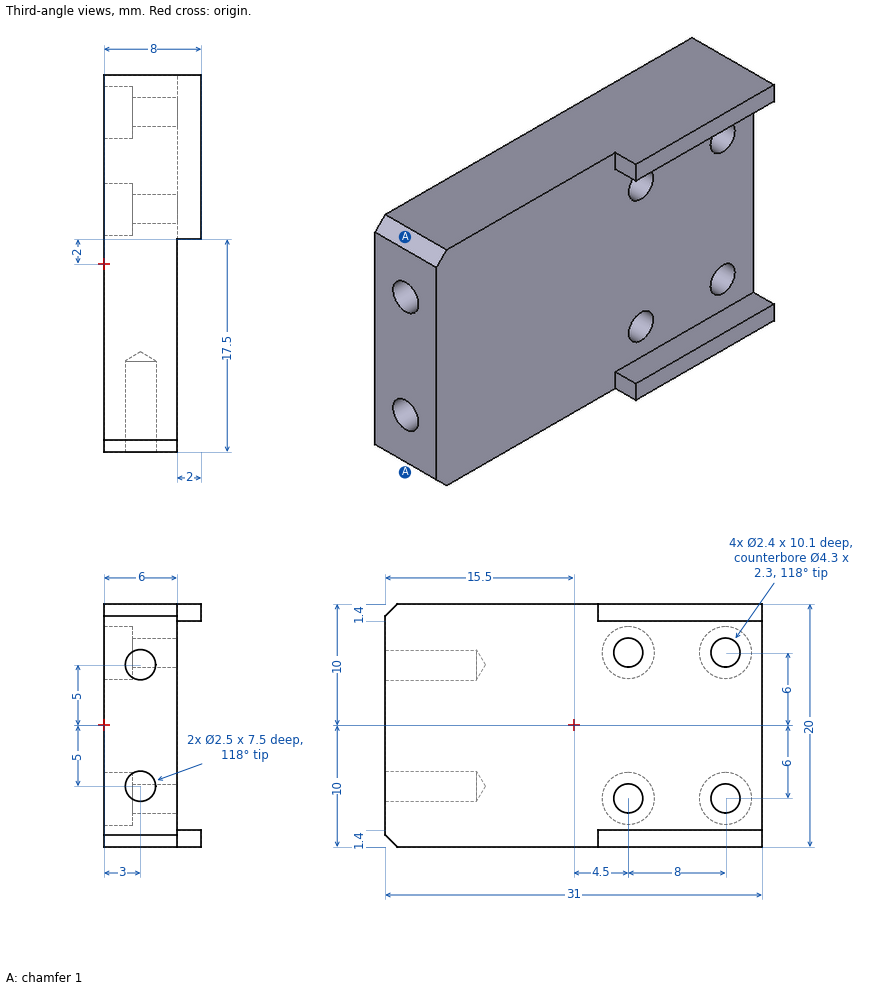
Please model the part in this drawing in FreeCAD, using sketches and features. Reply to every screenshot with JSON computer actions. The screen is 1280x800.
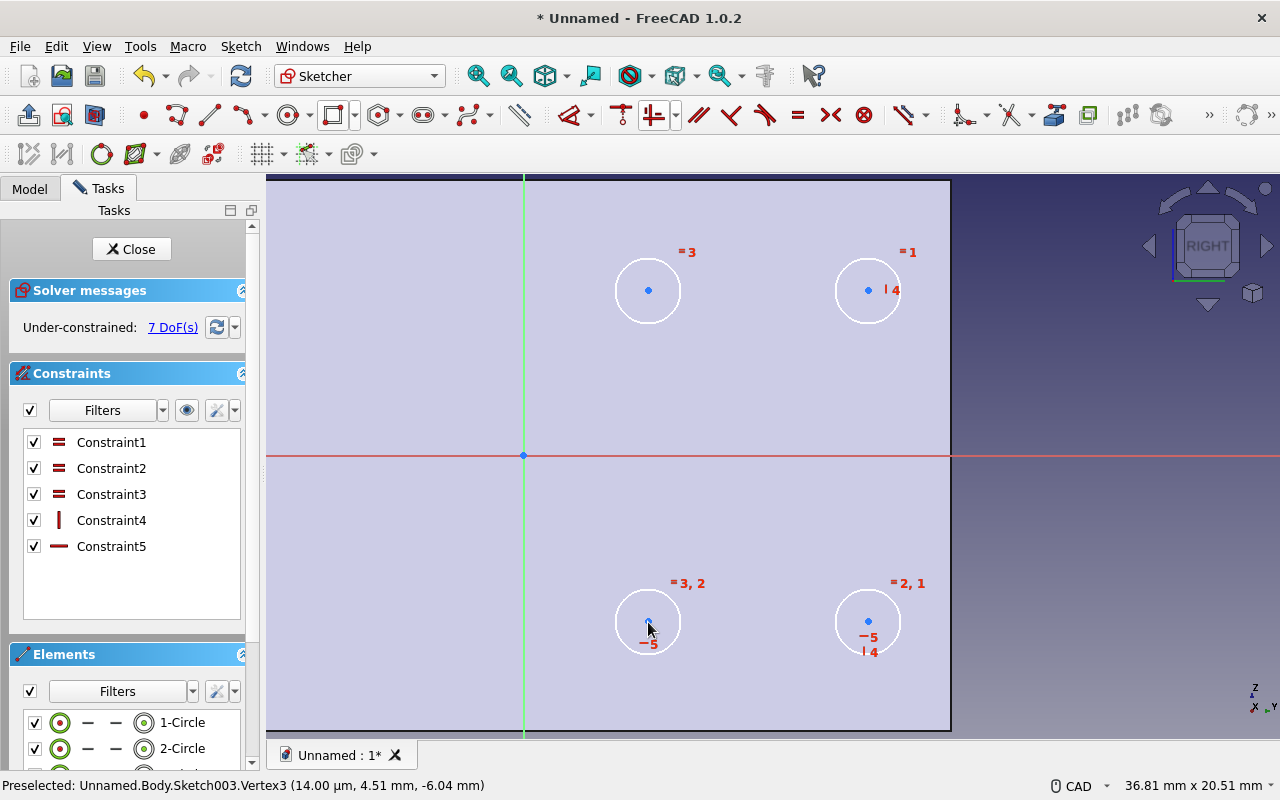
{"action": "left_click", "coordinate": [648, 622]}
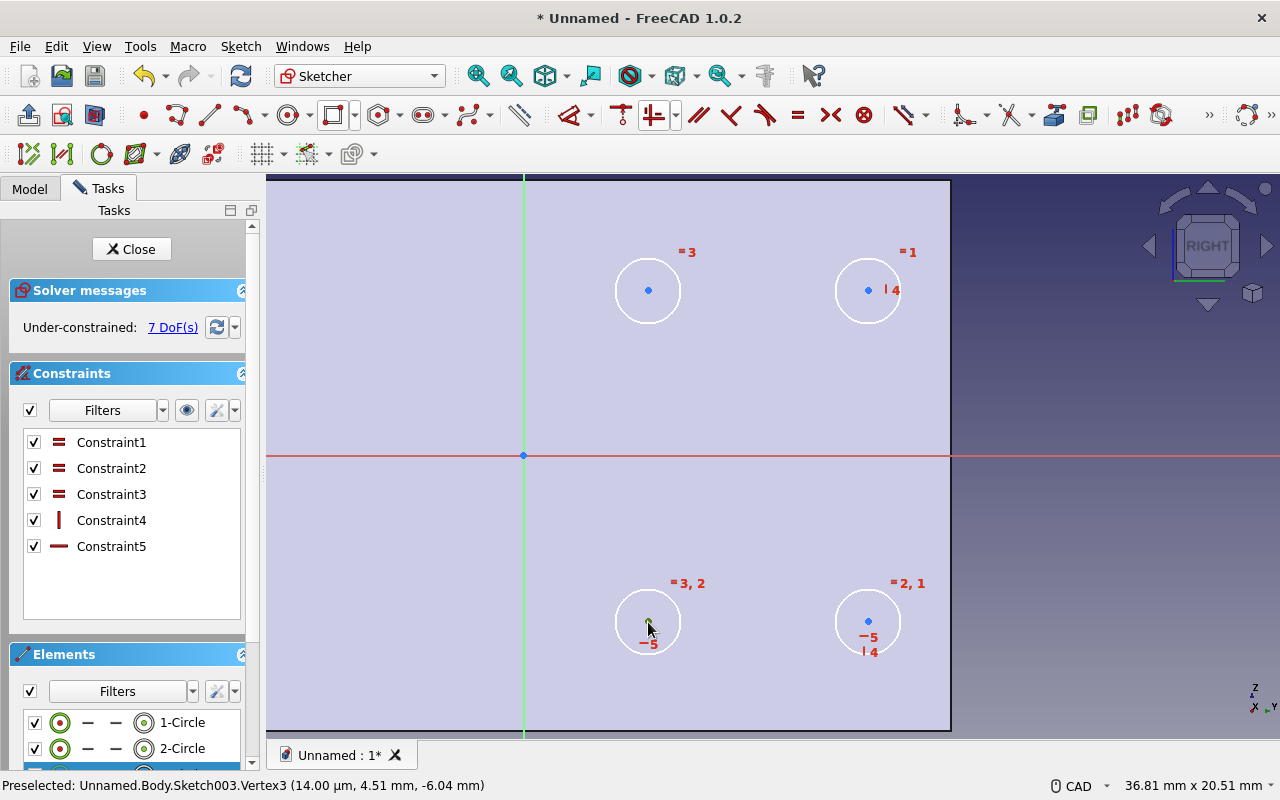
{"action": "left_click", "coordinate": [648, 291]}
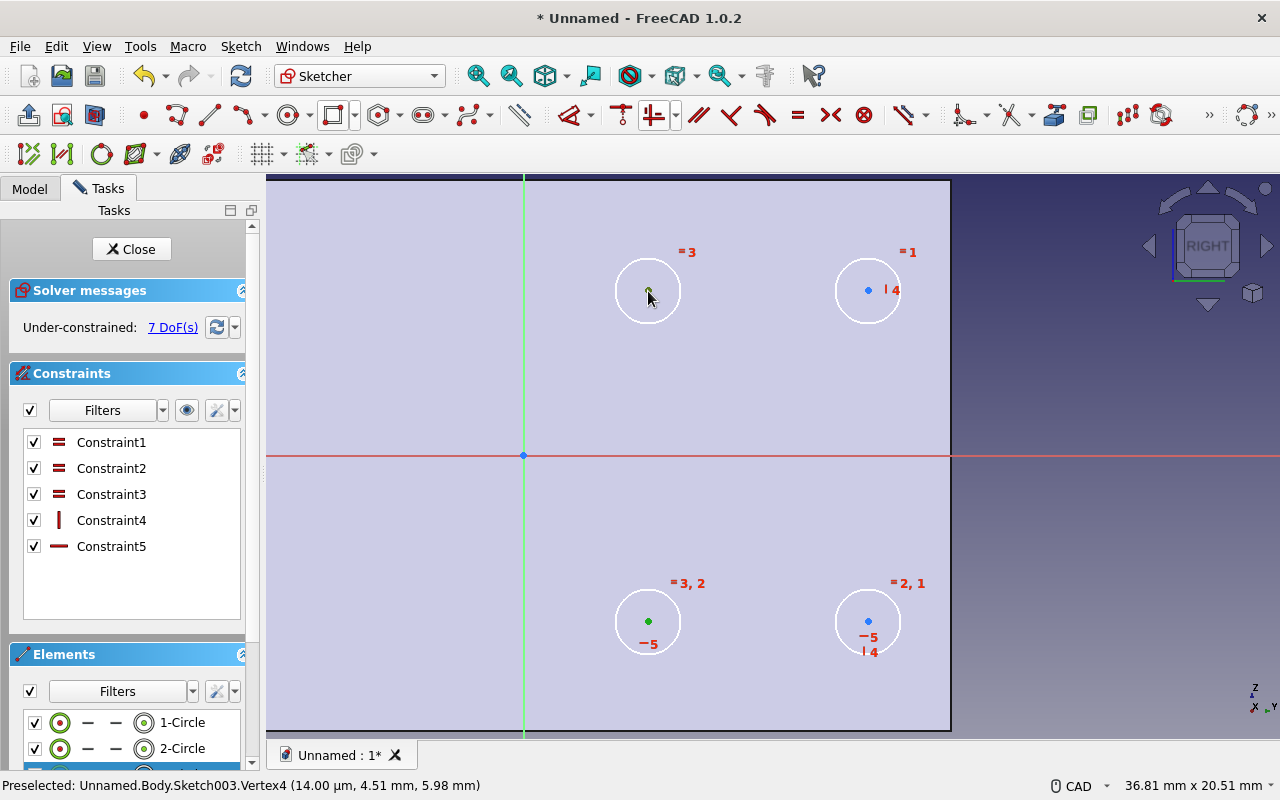
{"action": "key", "text": "v"}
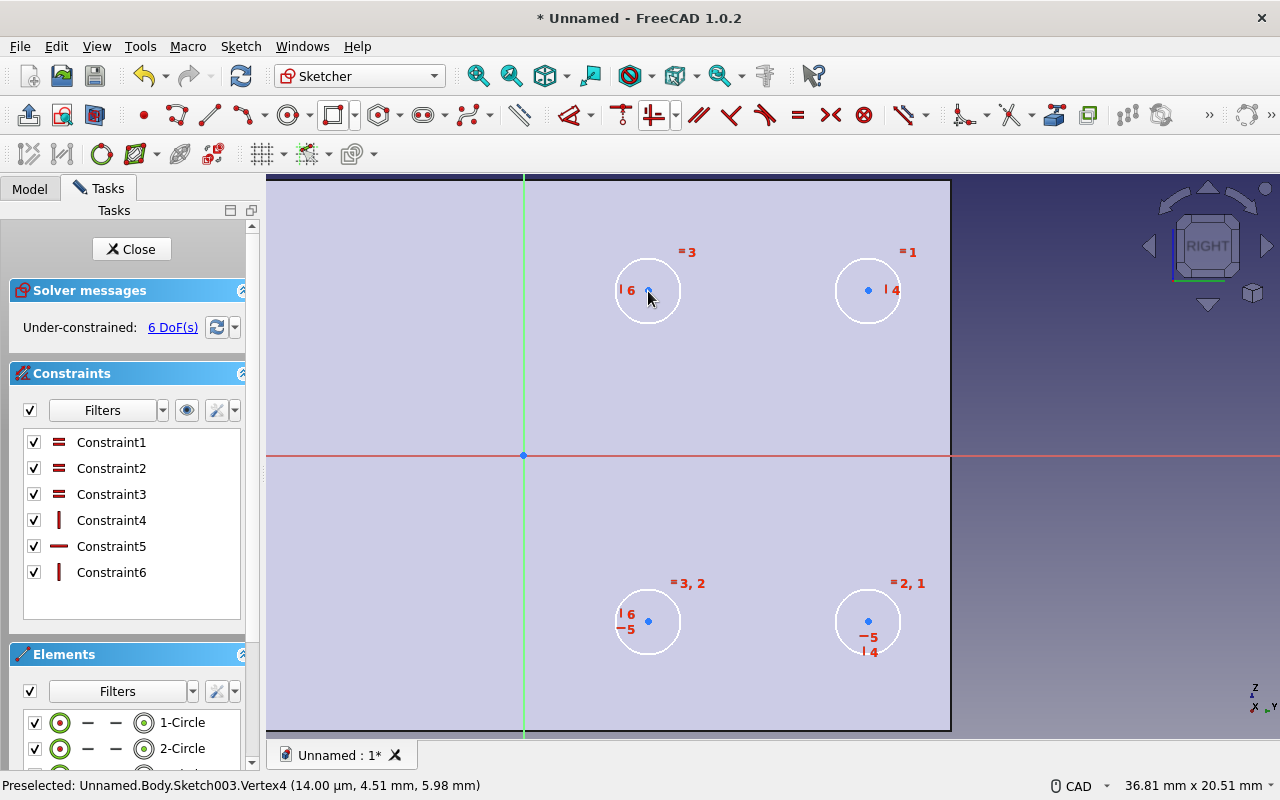
{"action": "left_click", "coordinate": [868, 291]}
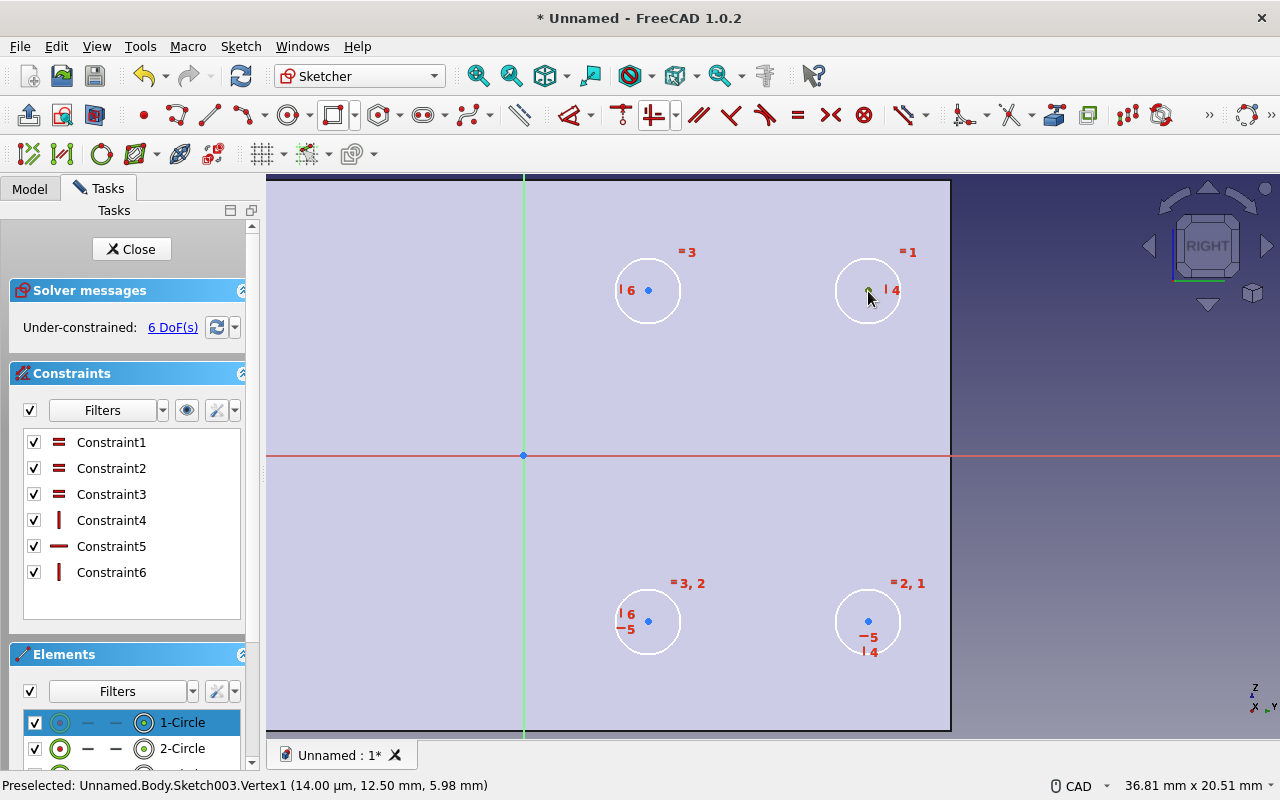
{"action": "left_click", "coordinate": [648, 291]}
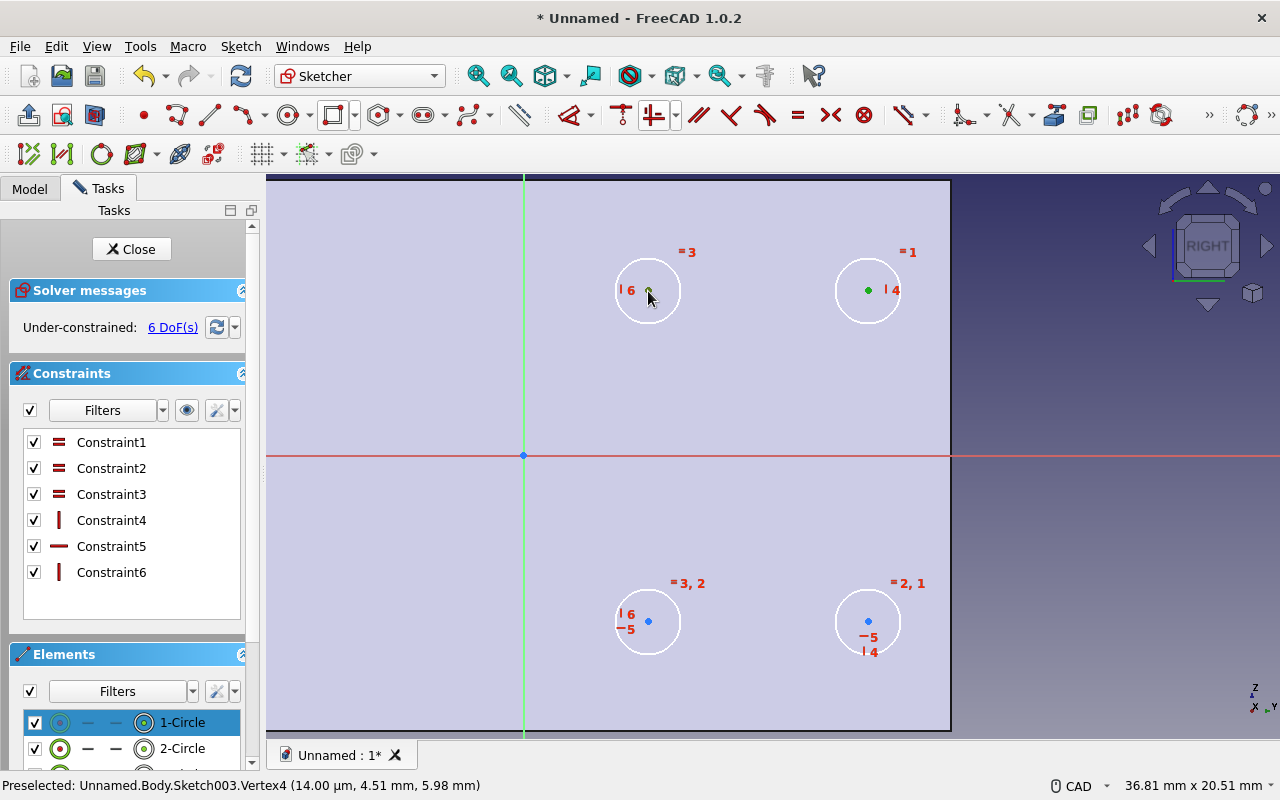
{"action": "left_click", "coordinate": [676, 116]}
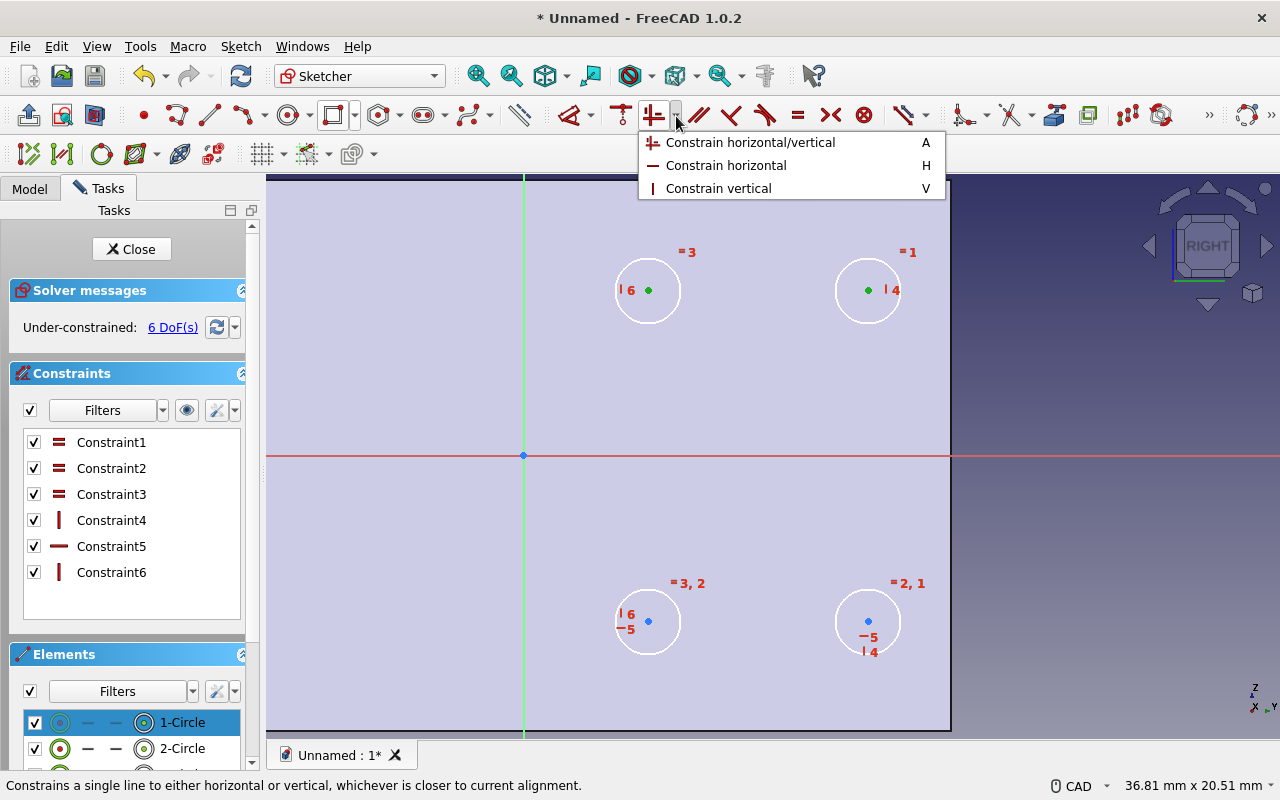
{"action": "left_click", "coordinate": [792, 166]}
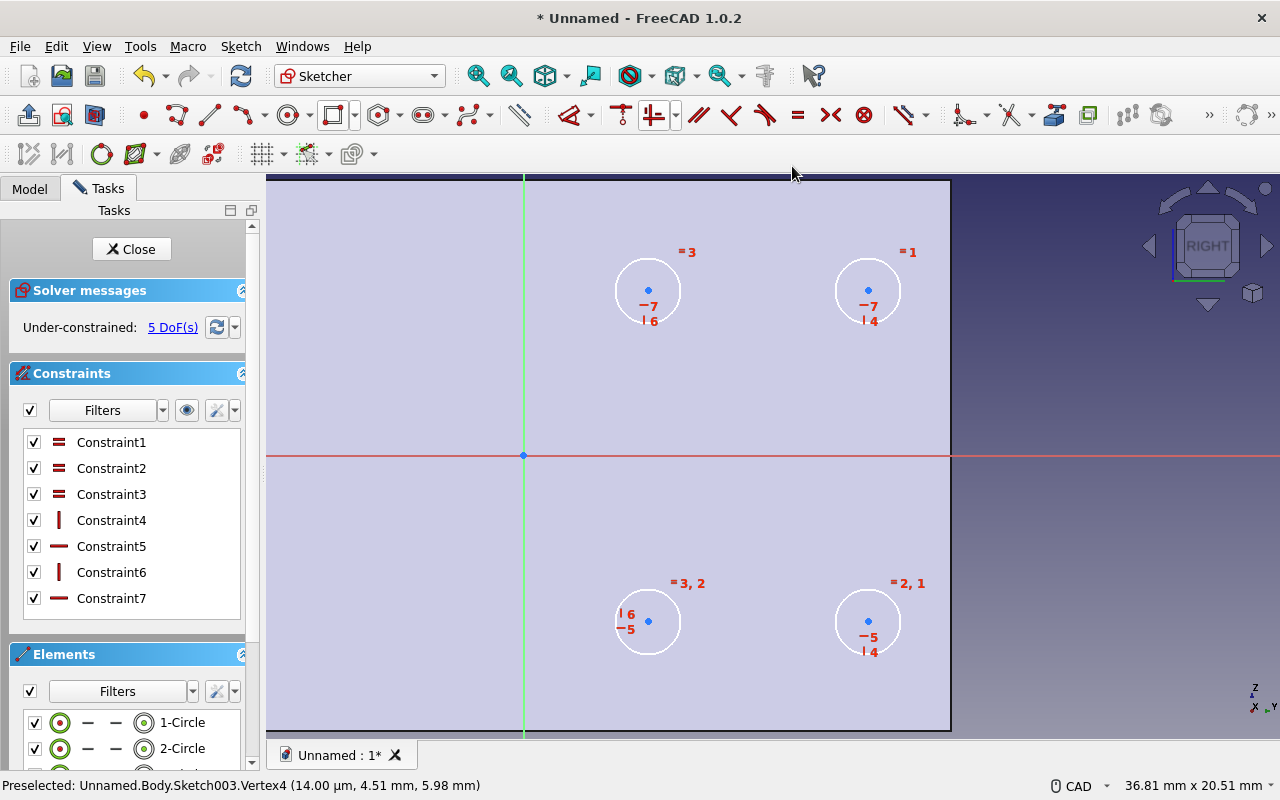
{"action": "left_click", "coordinate": [568, 116]}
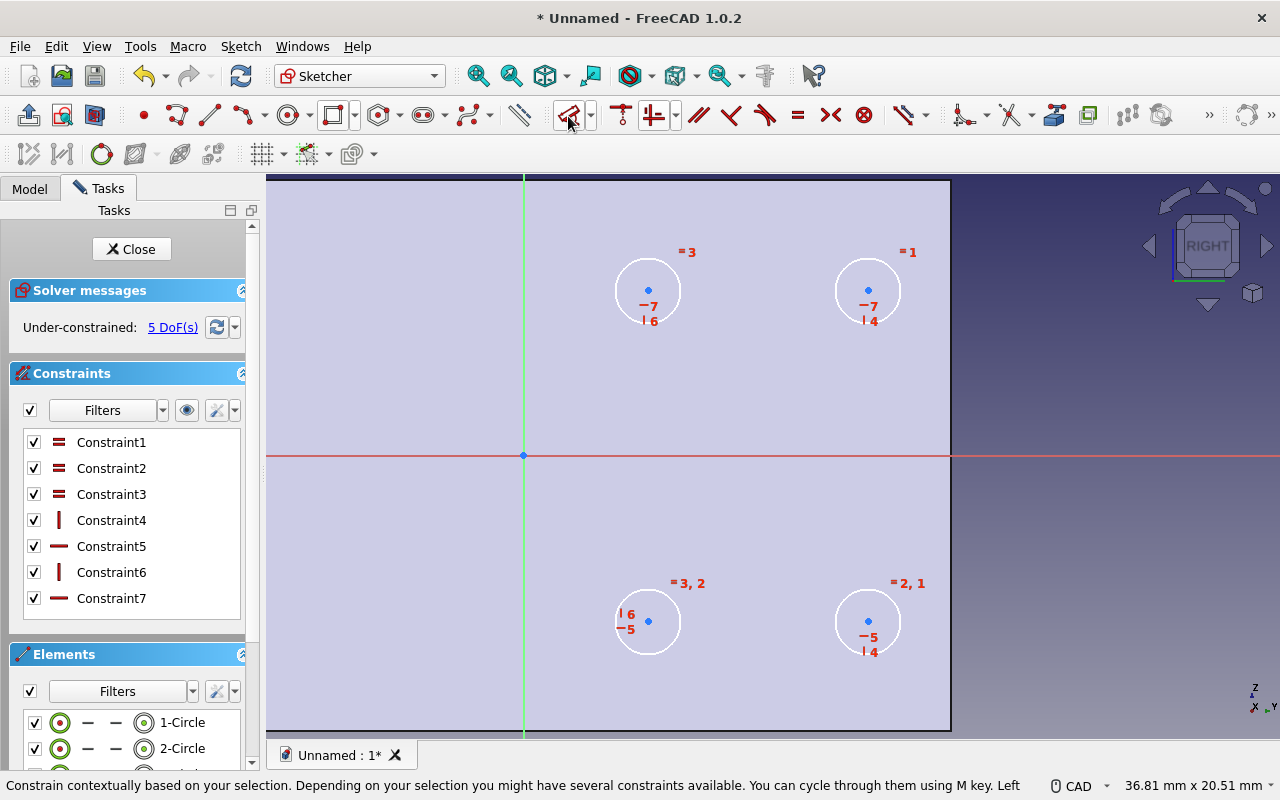
{"action": "left_click", "coordinate": [891, 268]}
{"action": "left_click", "coordinate": [914, 245]}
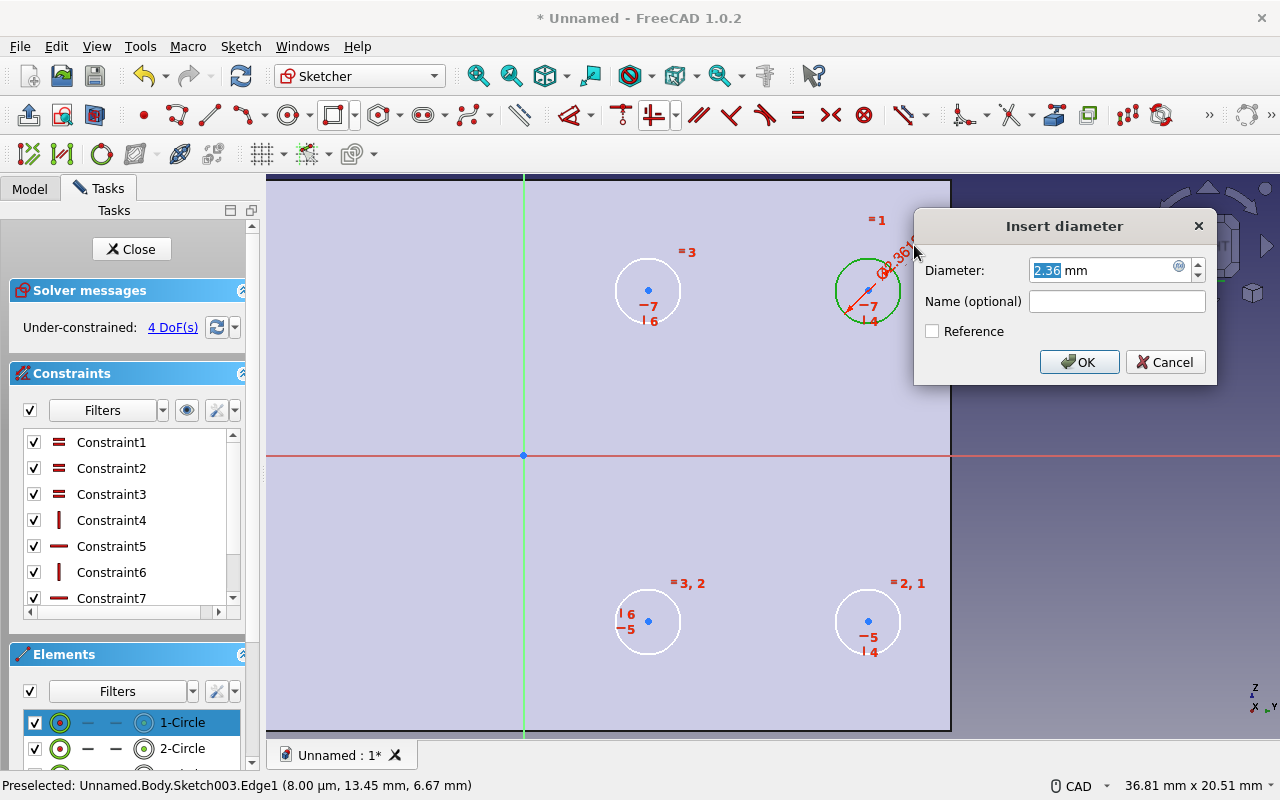
{"action": "type", "text": "2.4"}
{"action": "key", "text": "Return"}